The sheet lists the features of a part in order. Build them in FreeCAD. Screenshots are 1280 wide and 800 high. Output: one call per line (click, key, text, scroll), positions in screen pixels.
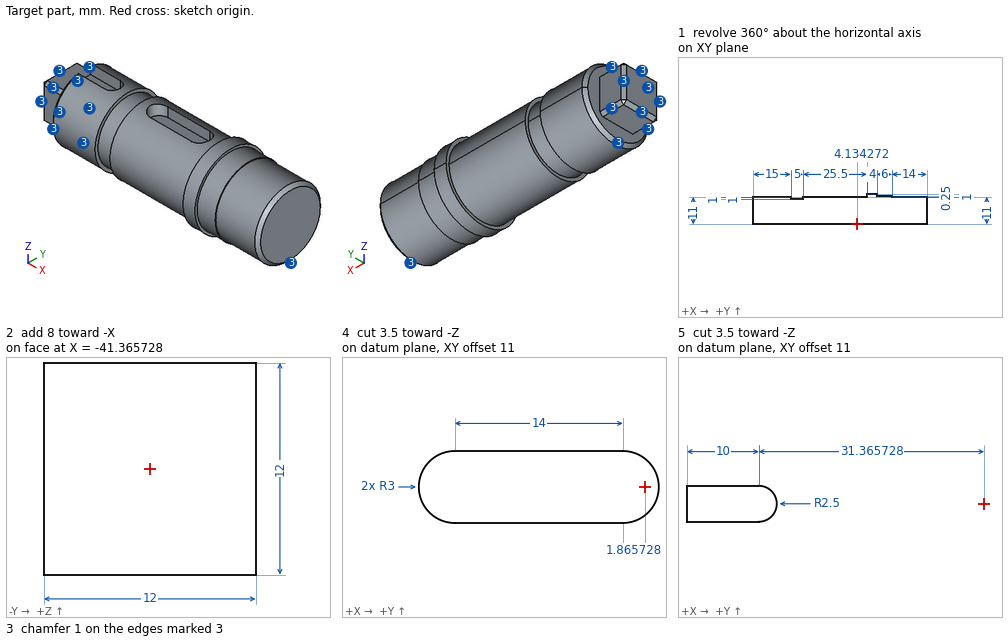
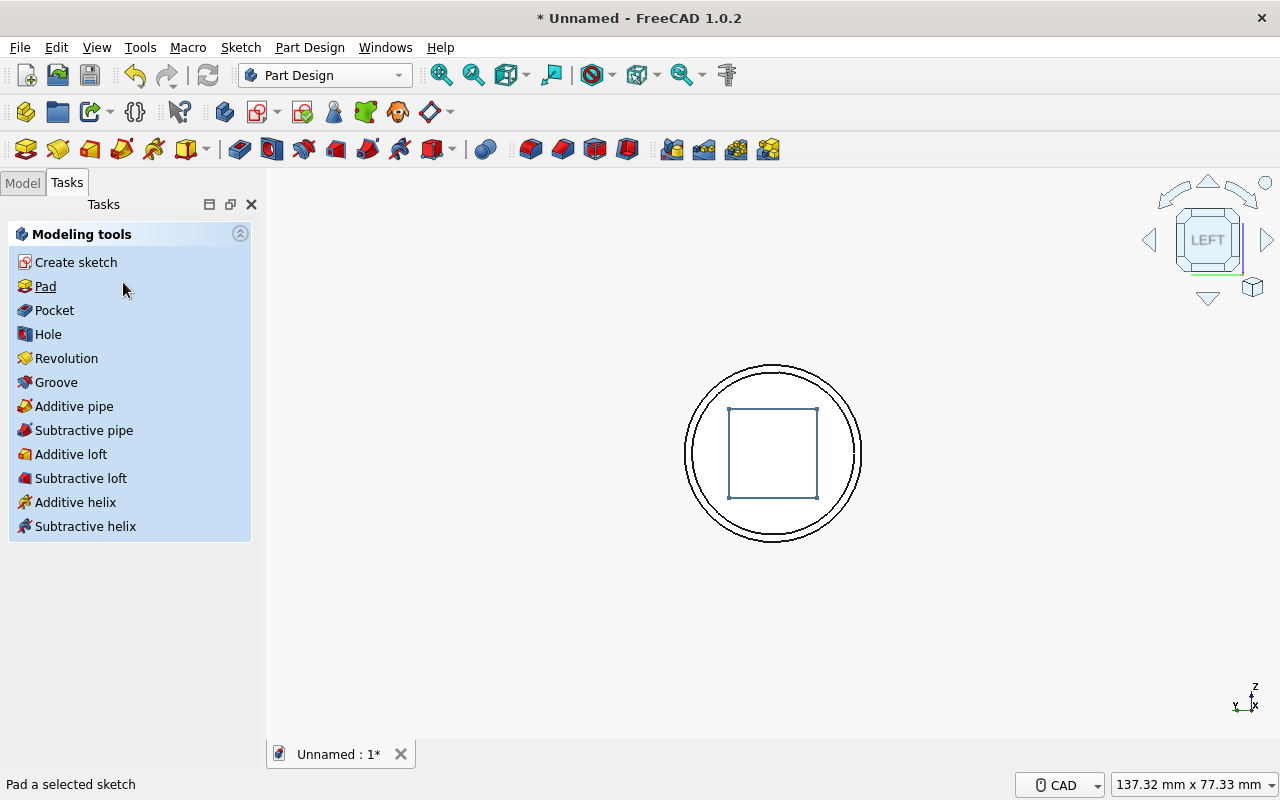
click(26, 150)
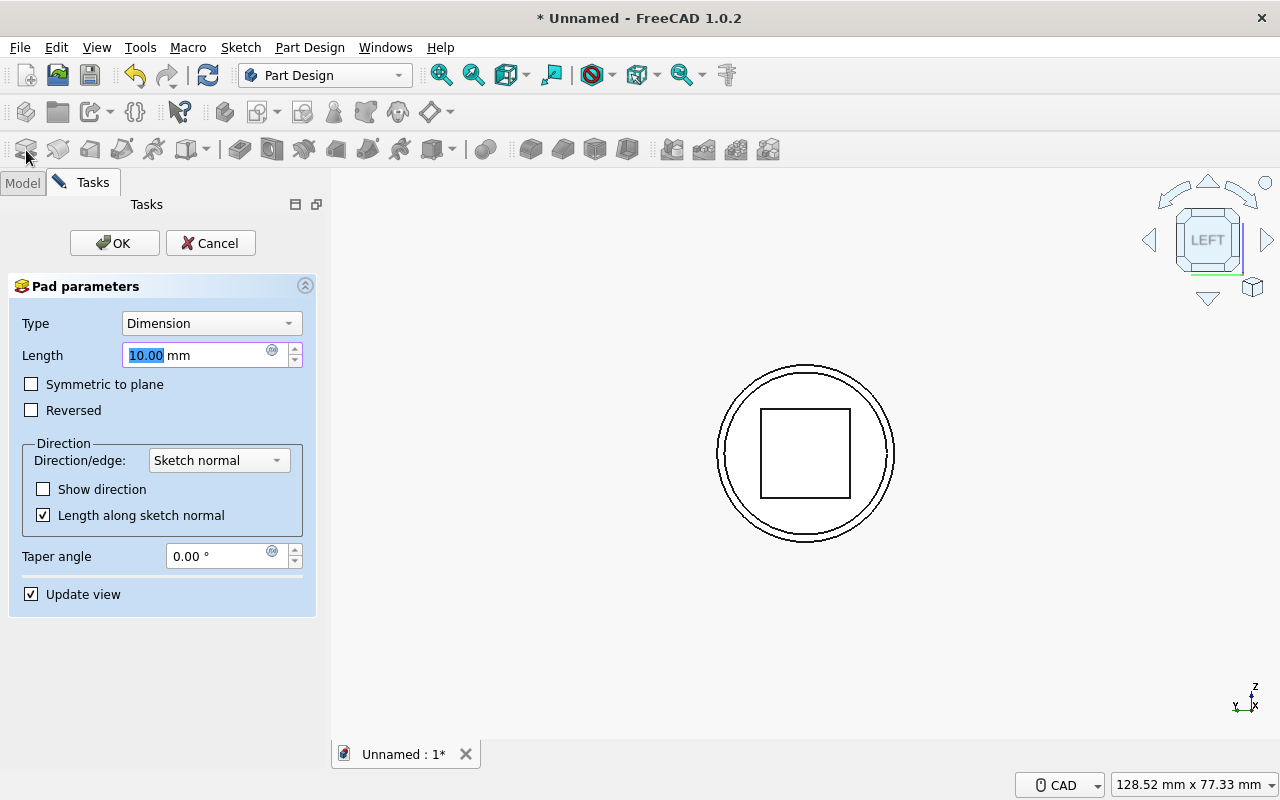
text(8)
key(Tab)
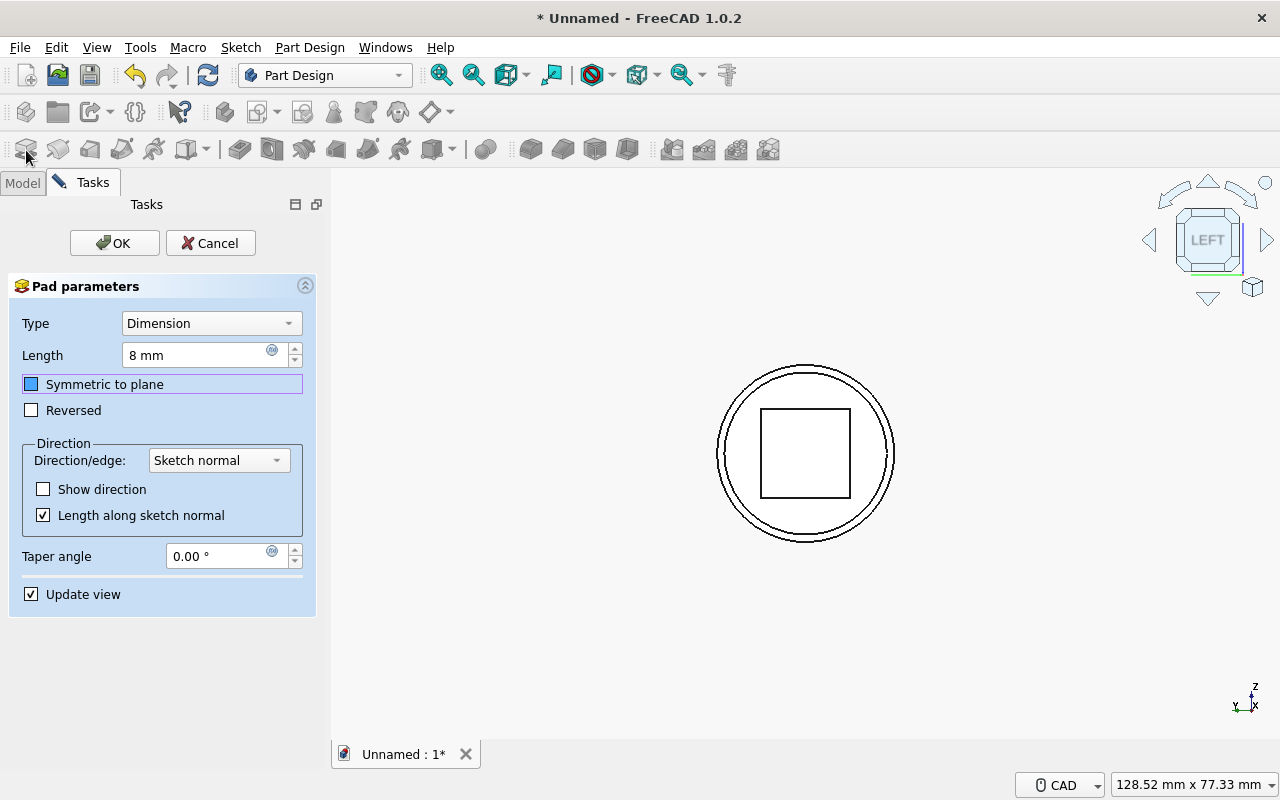
click(115, 243)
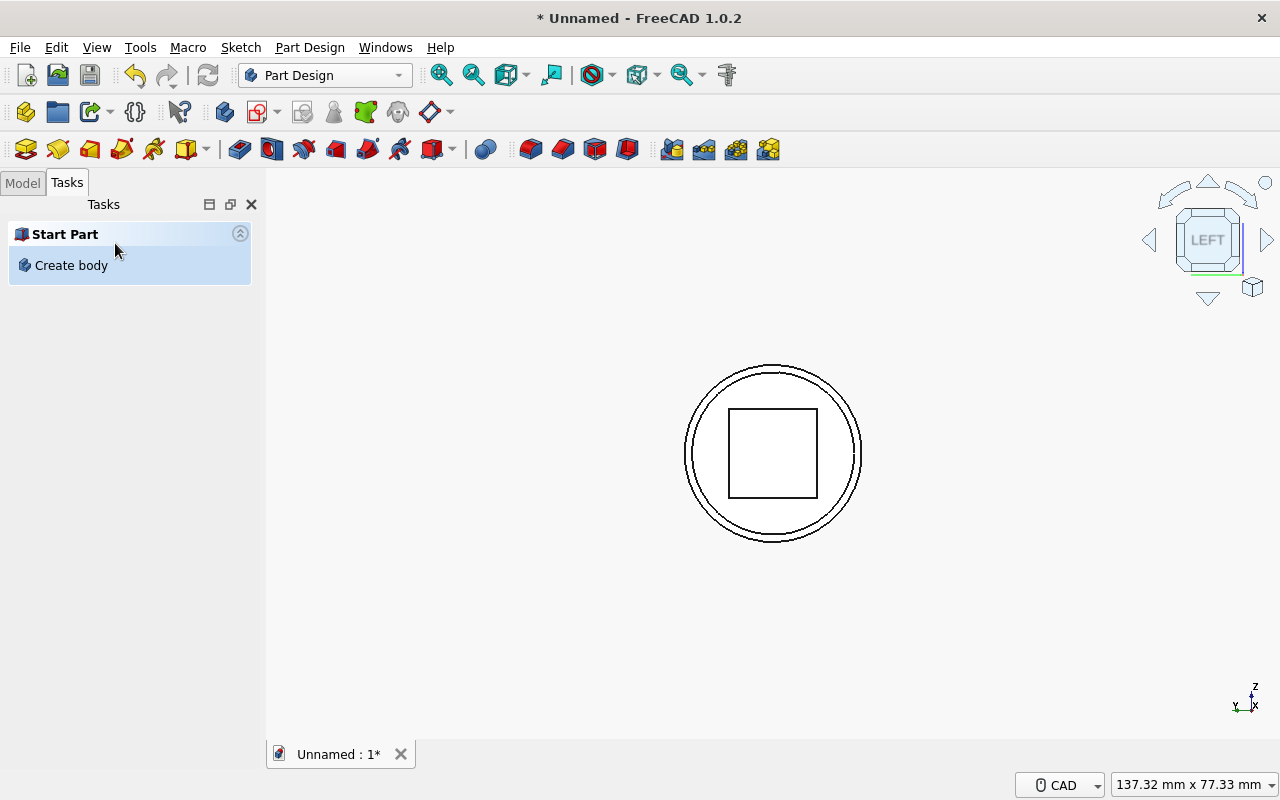
click(442, 76)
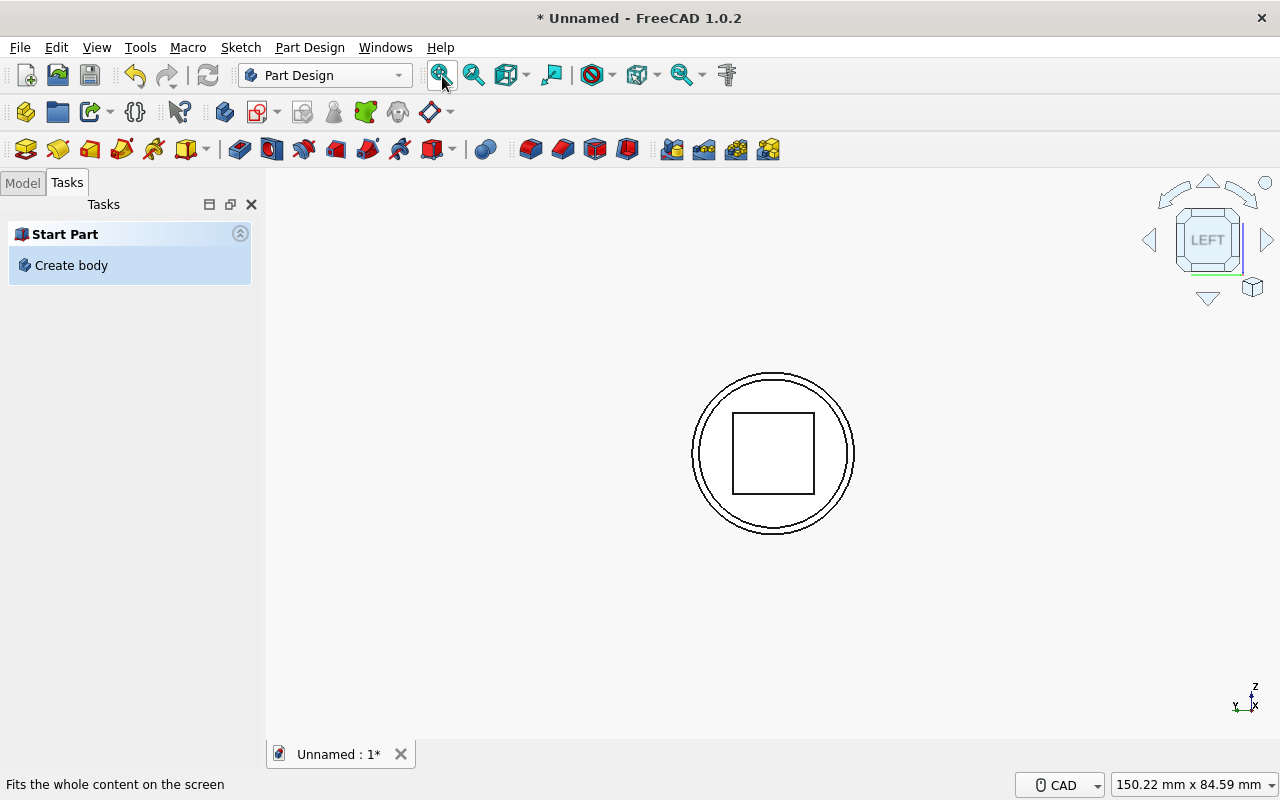
click(773, 452)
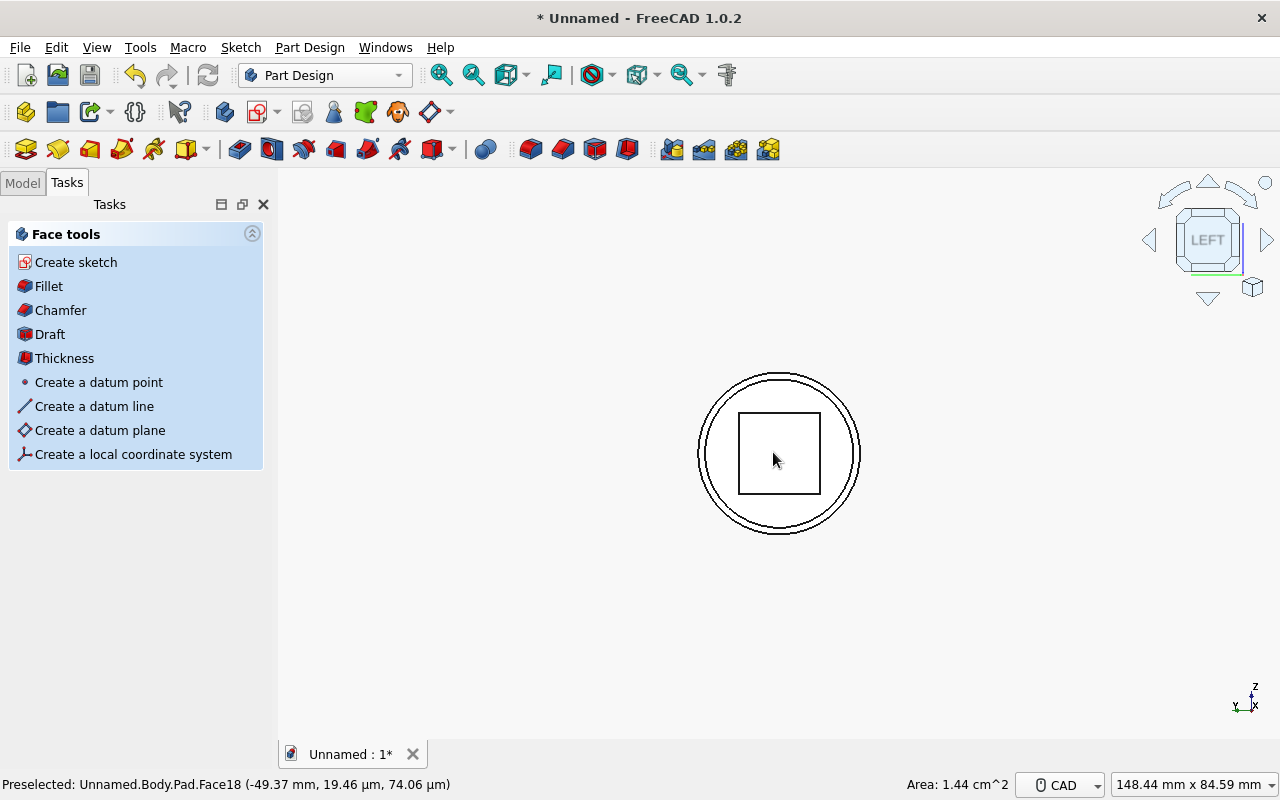
click(853, 452, ctrl)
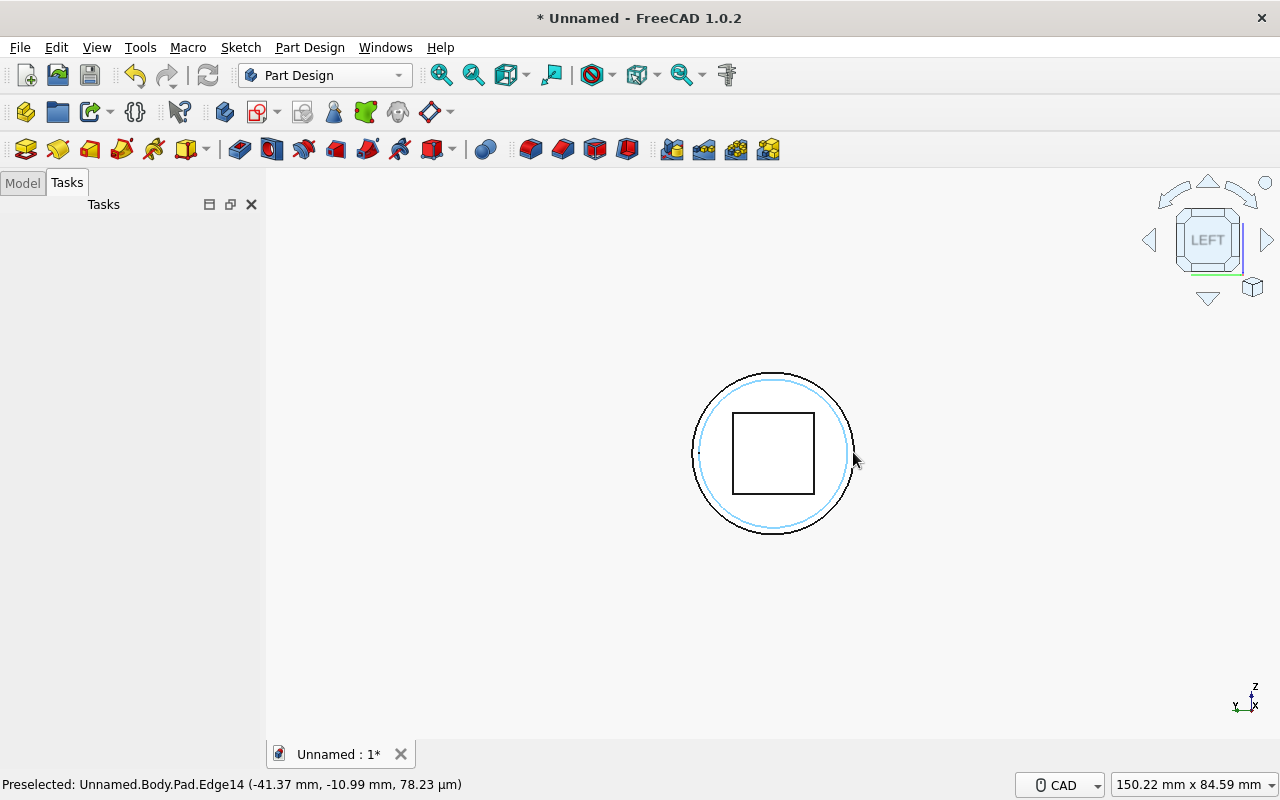
key(0)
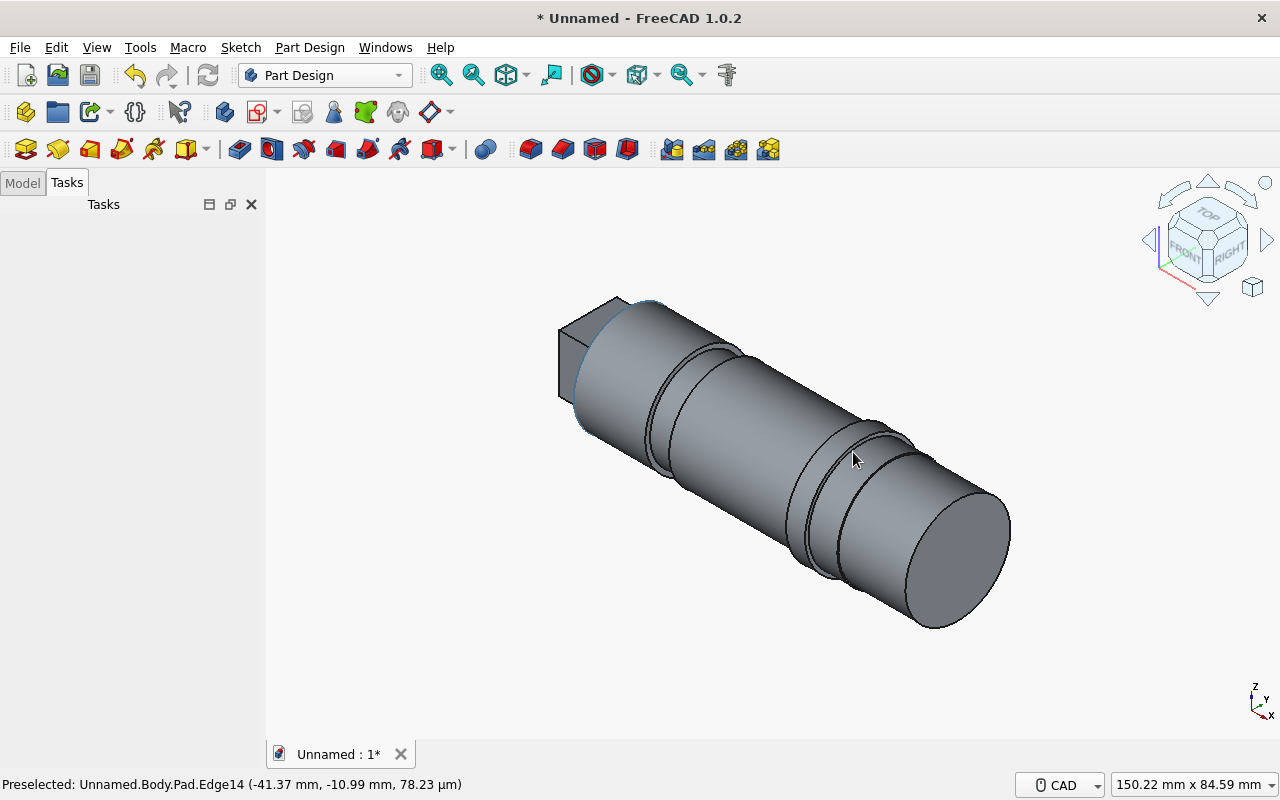
click(905, 590, ctrl)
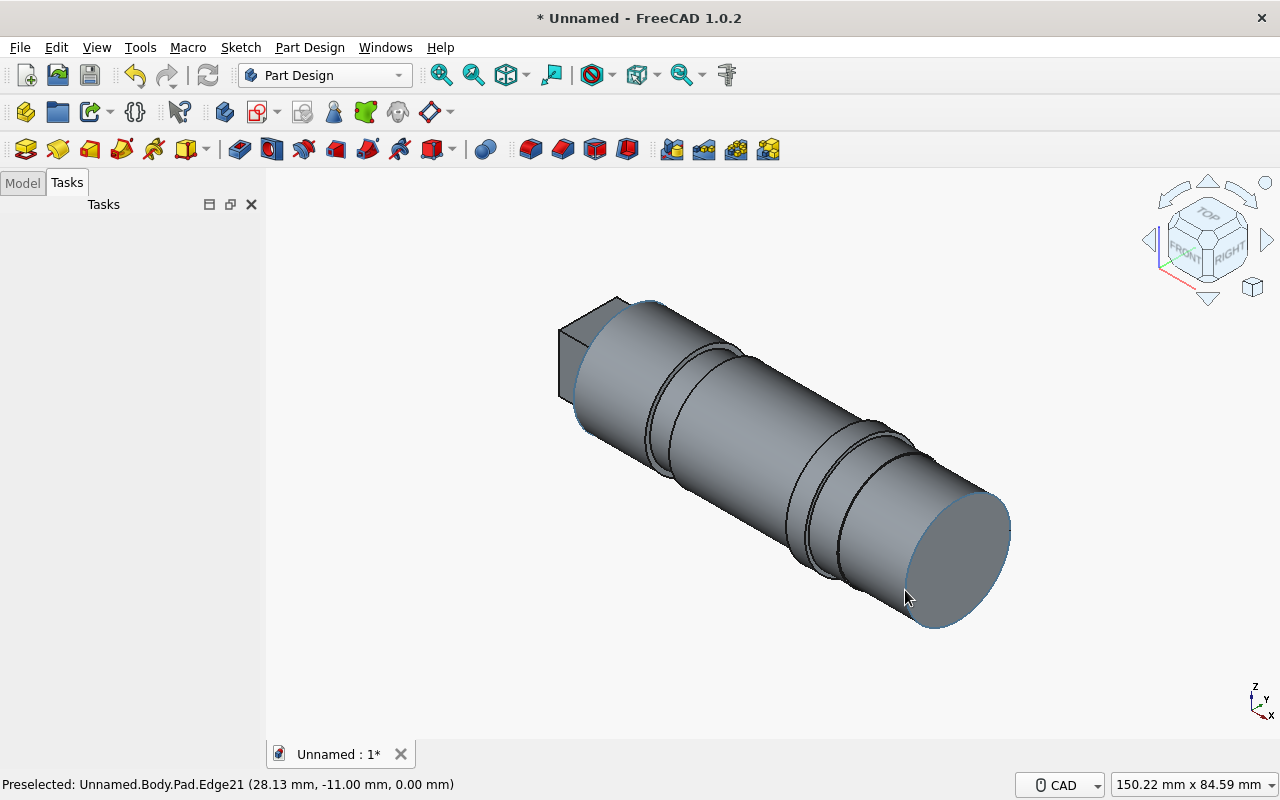
click(578, 340, ctrl)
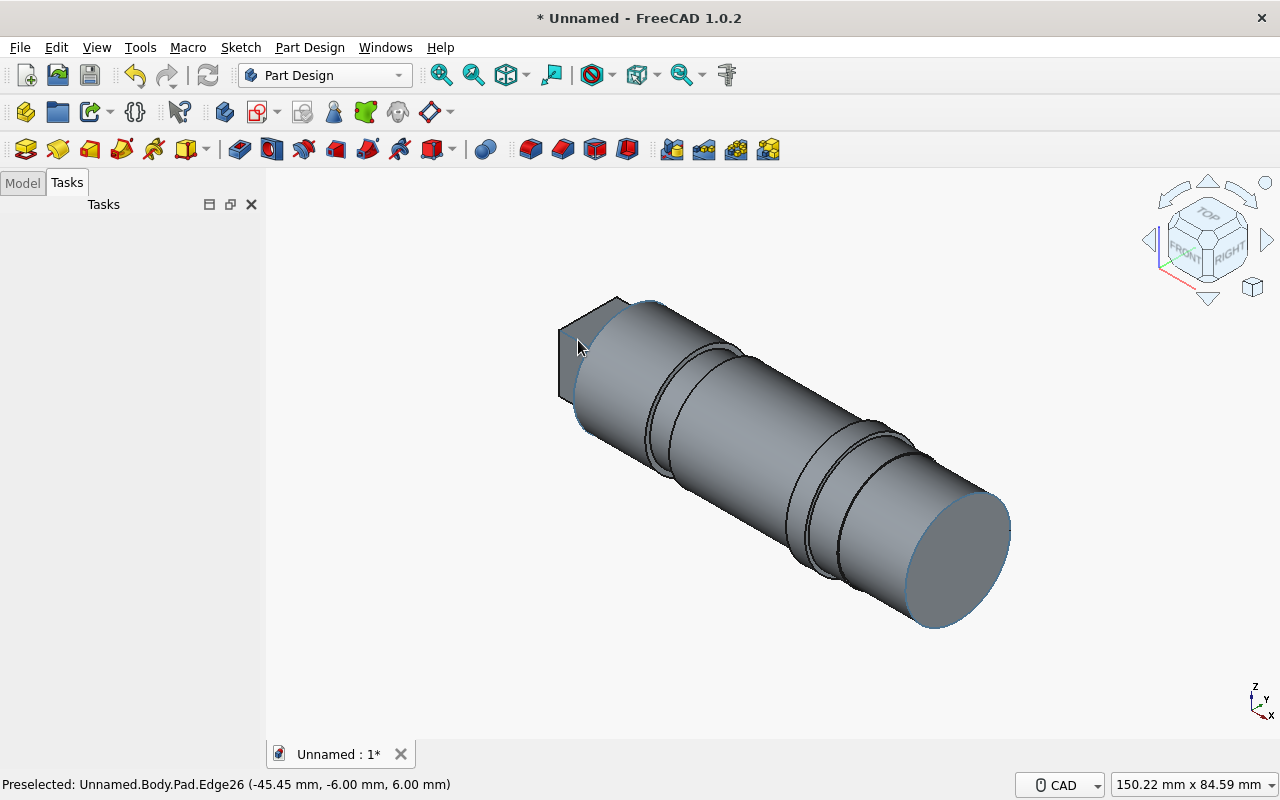
key(2)